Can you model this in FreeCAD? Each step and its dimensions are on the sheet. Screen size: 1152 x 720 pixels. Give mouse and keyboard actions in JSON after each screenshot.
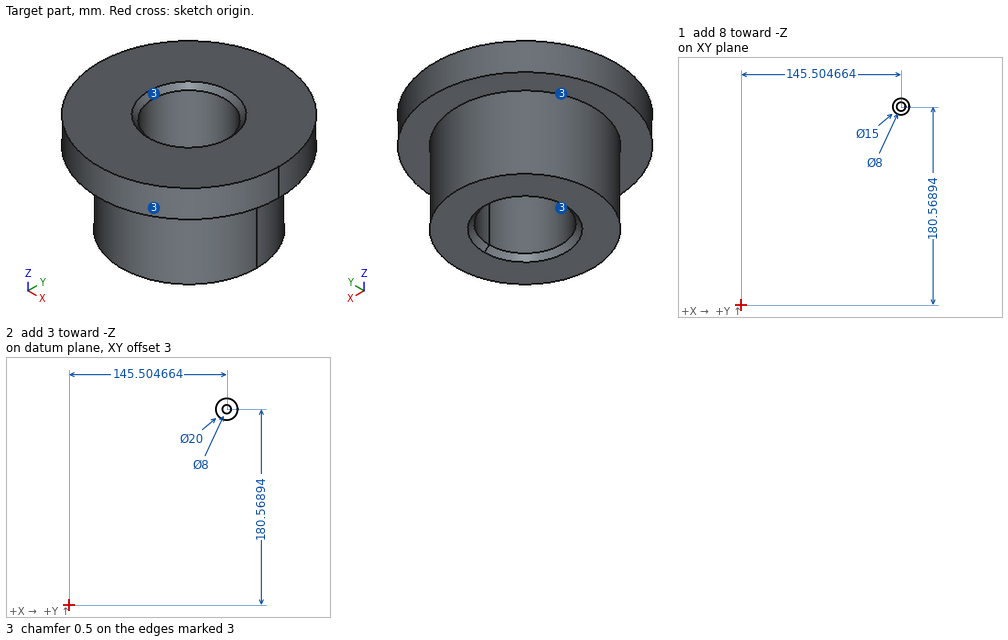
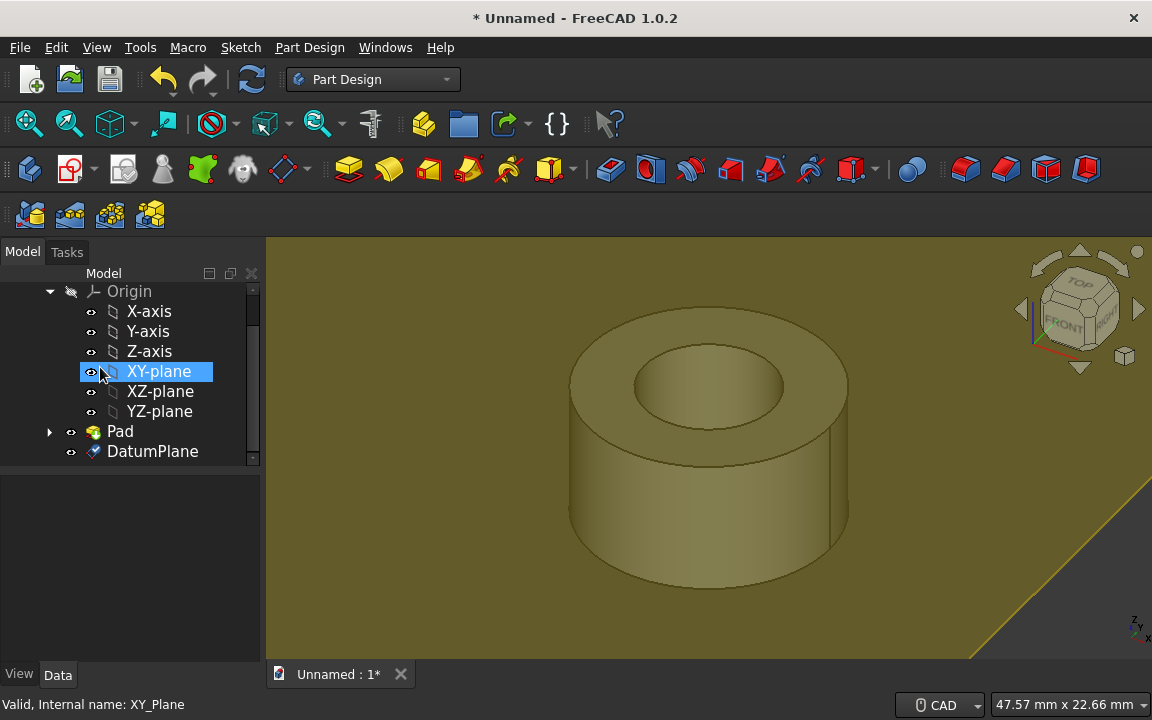
{"action": "left_click", "coordinate": [116, 452]}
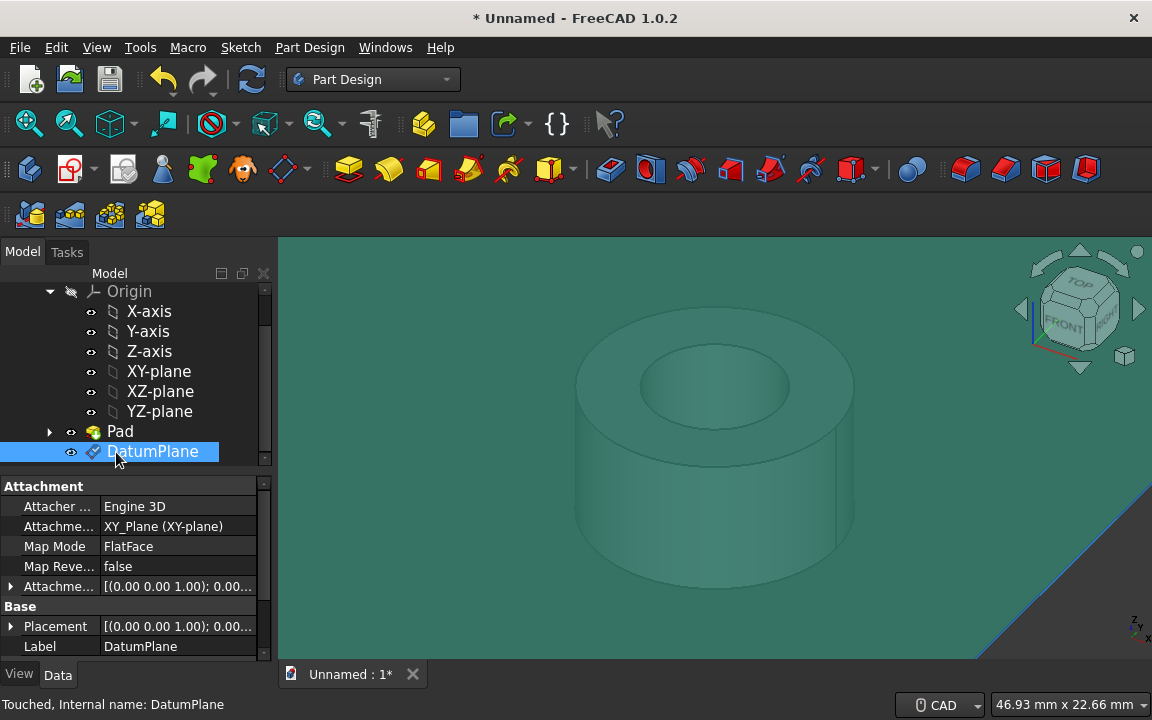
{"action": "left_click", "coordinate": [70, 170]}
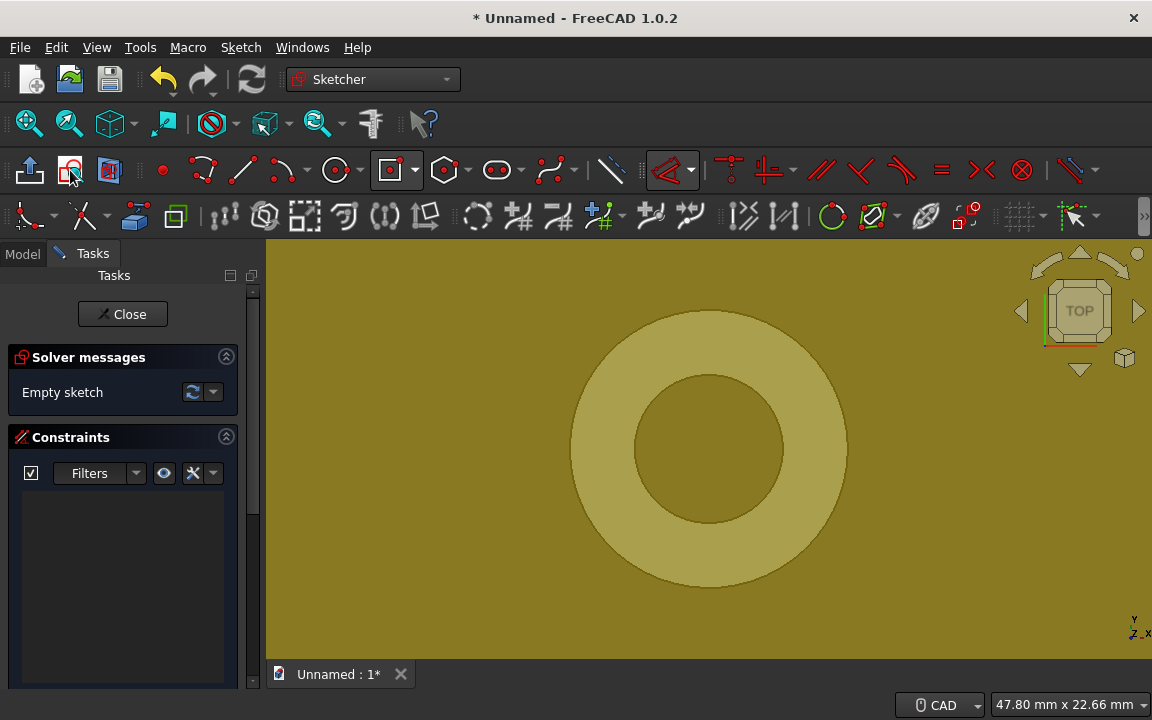
{"action": "scroll", "coordinate": [501, 449], "scroll_direction": "down", "scroll_amount": 2}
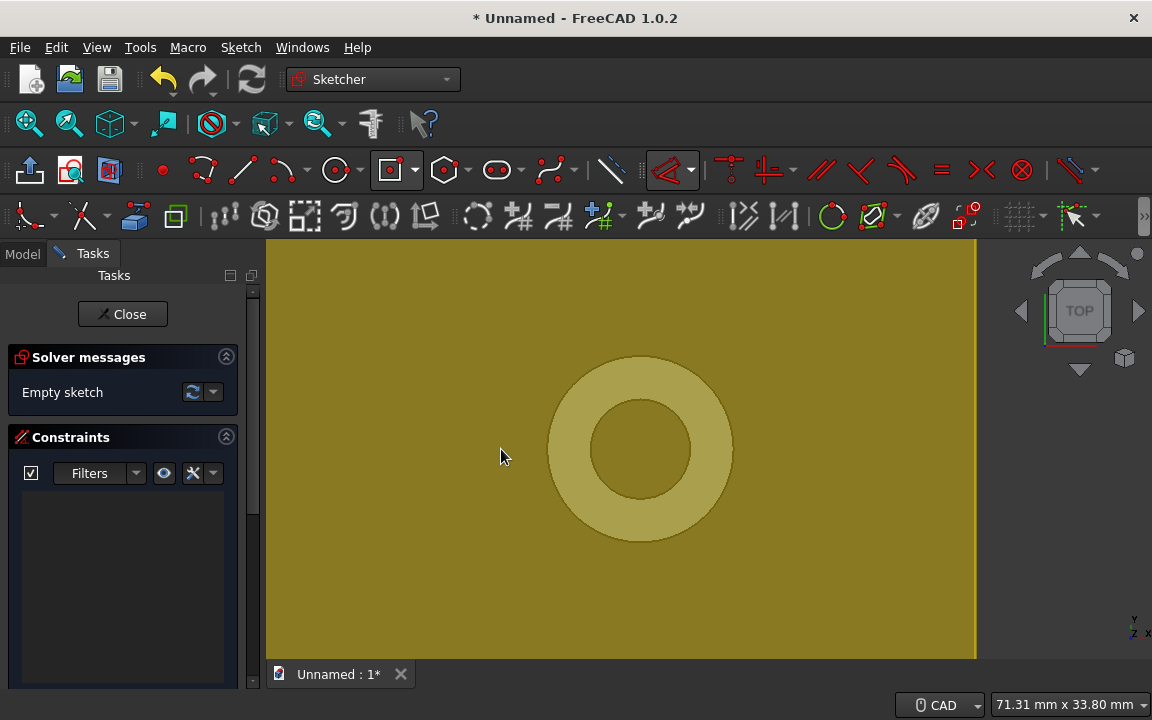
{"action": "key", "text": "g c"}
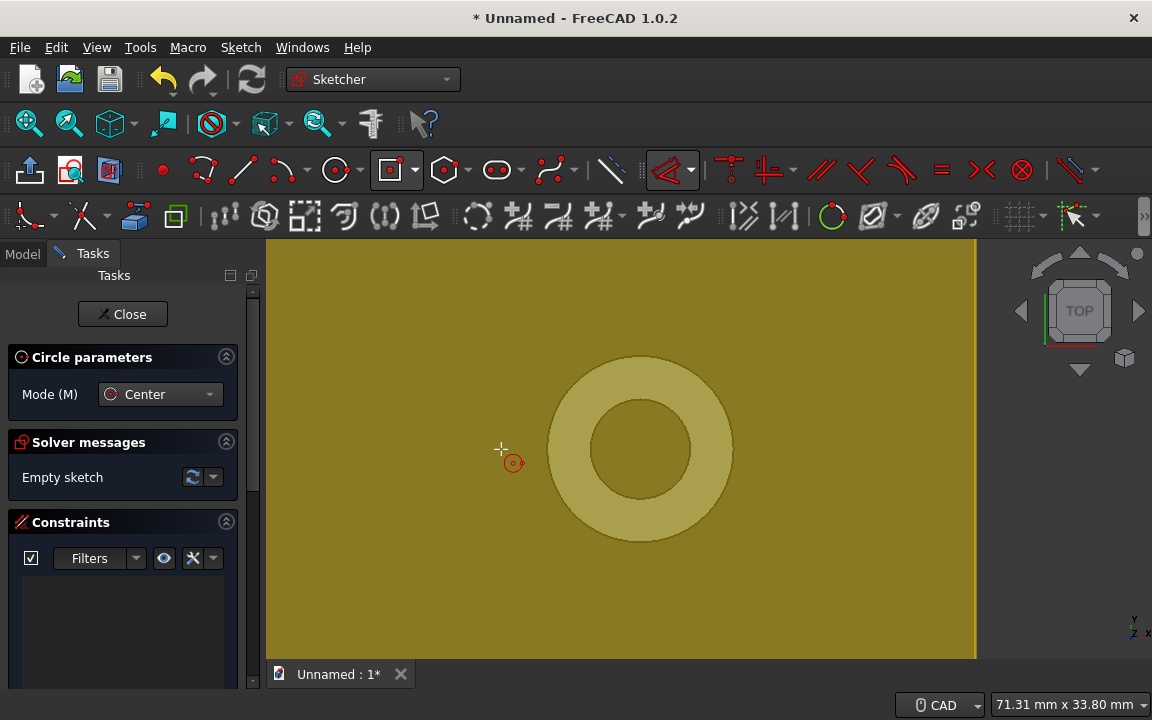
{"action": "left_click", "coordinate": [640, 449]}
{"action": "left_click", "coordinate": [728, 361]}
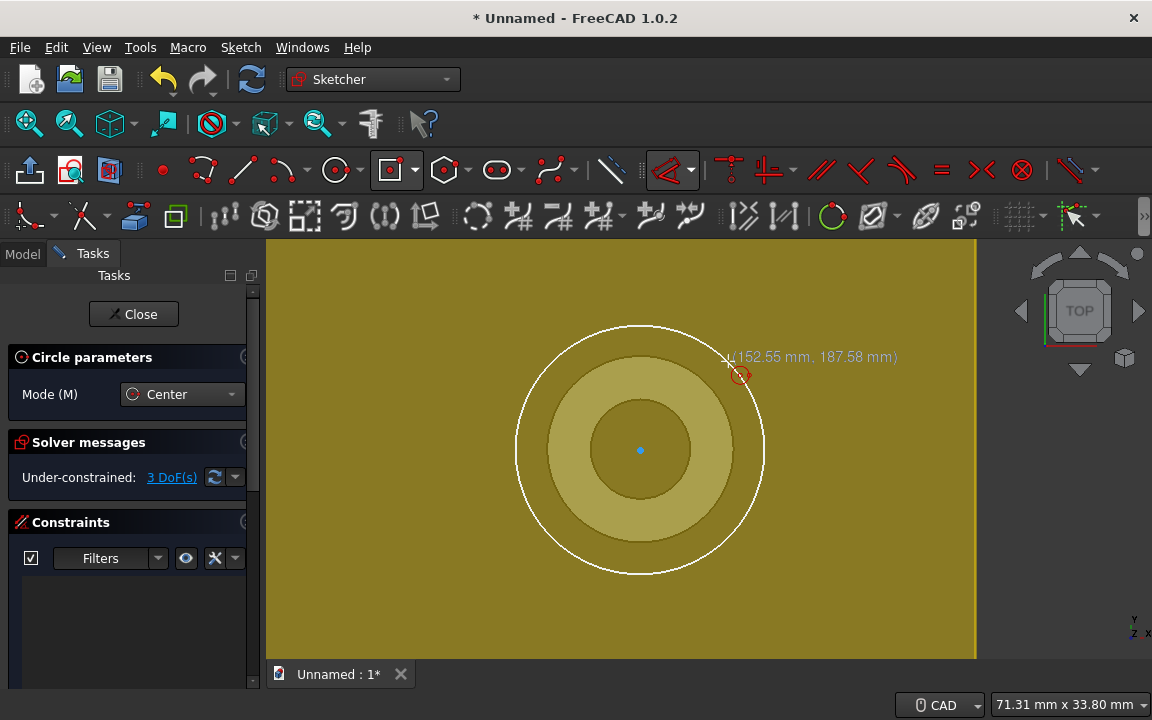
{"action": "left_click", "coordinate": [640, 450]}
{"action": "left_click", "coordinate": [676, 414]}
{"action": "key", "text": "Escape"}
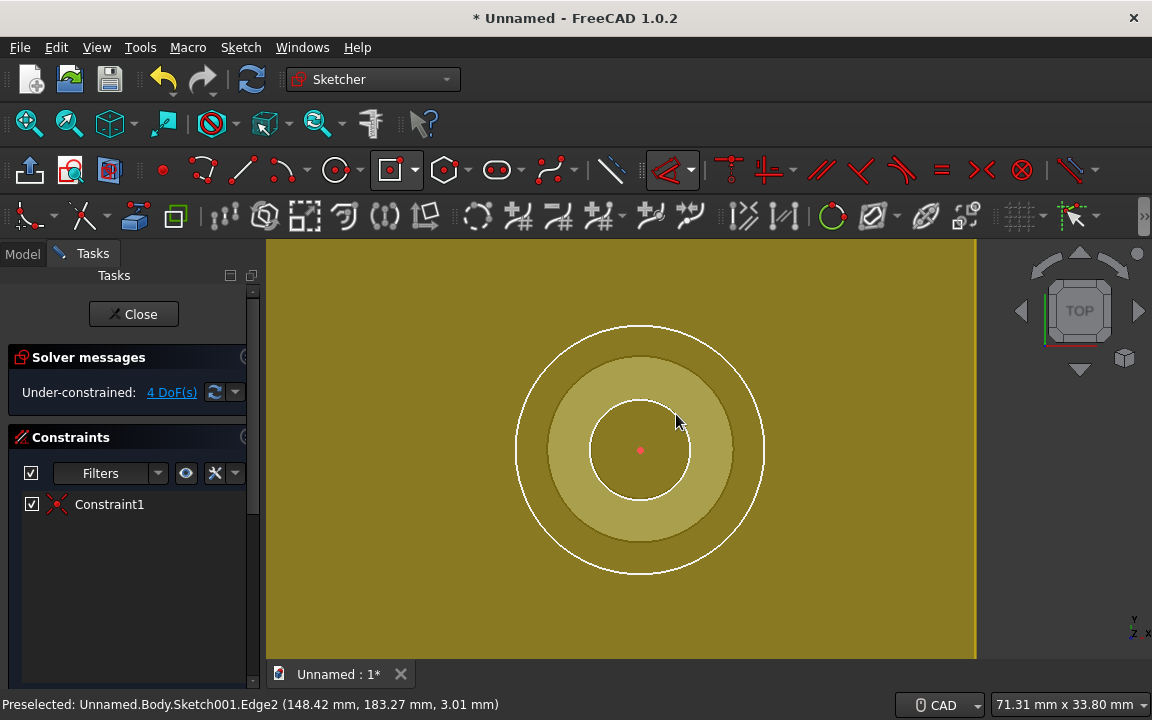
{"action": "key", "text": "d"}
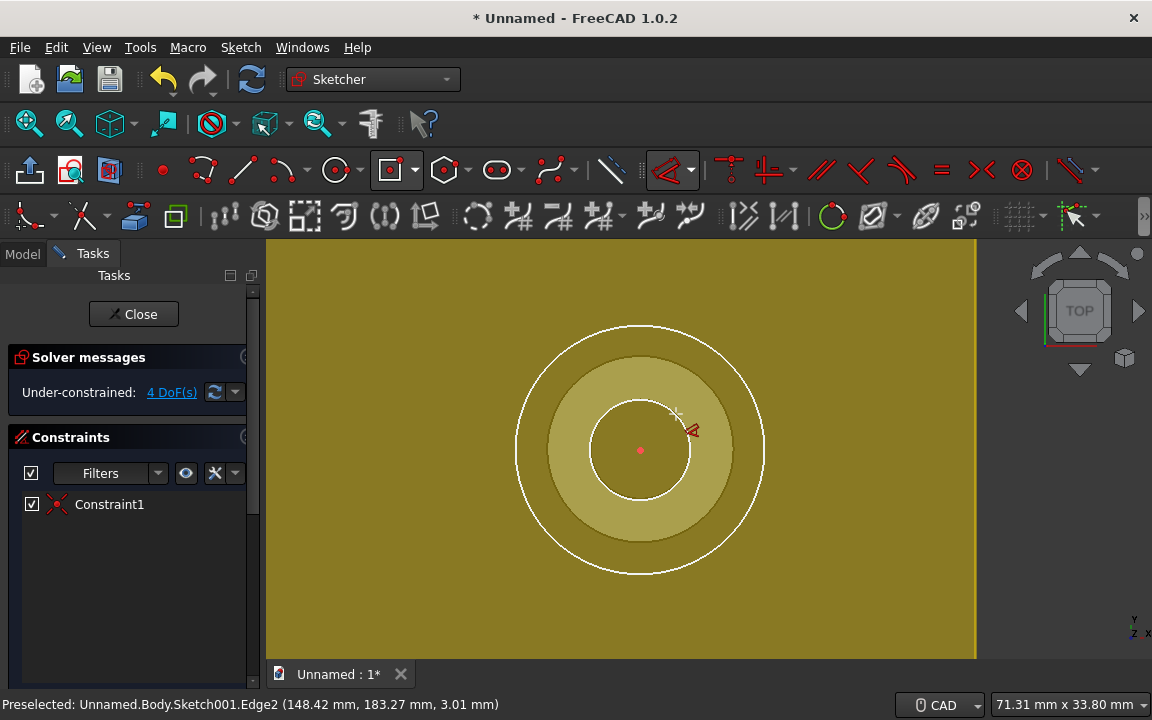
{"action": "left_click", "coordinate": [728, 362]}
{"action": "left_click", "coordinate": [751, 339]}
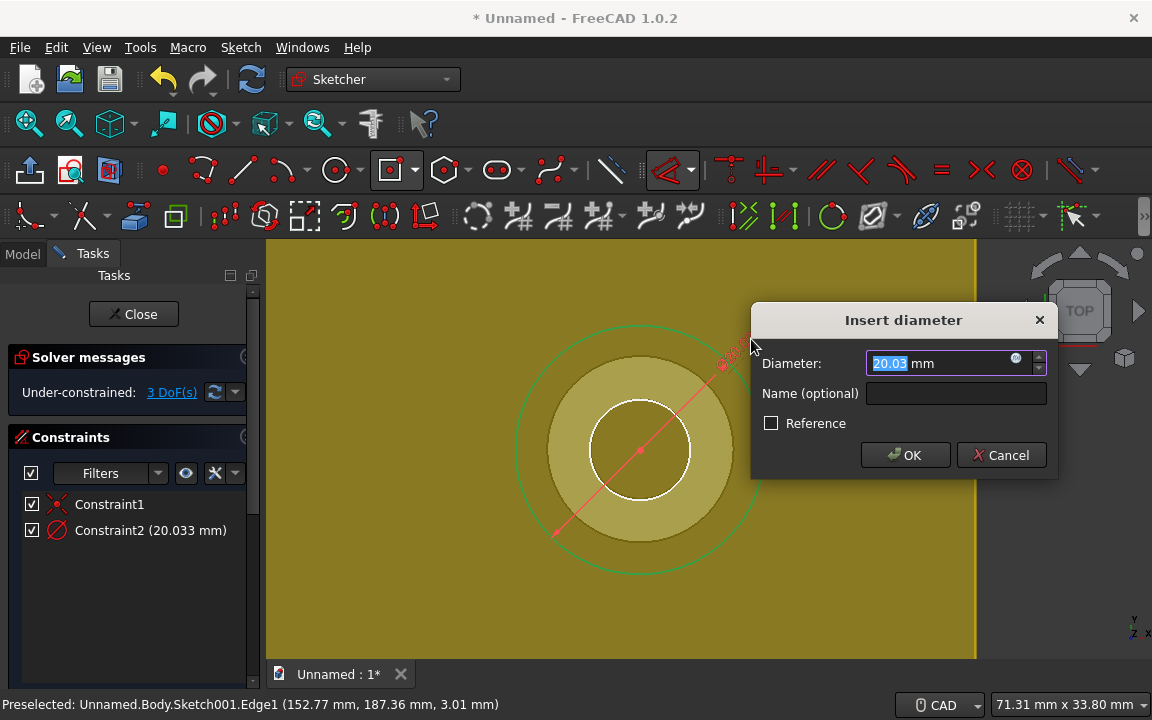
{"action": "type", "text": "20"}
{"action": "key", "text": "Return"}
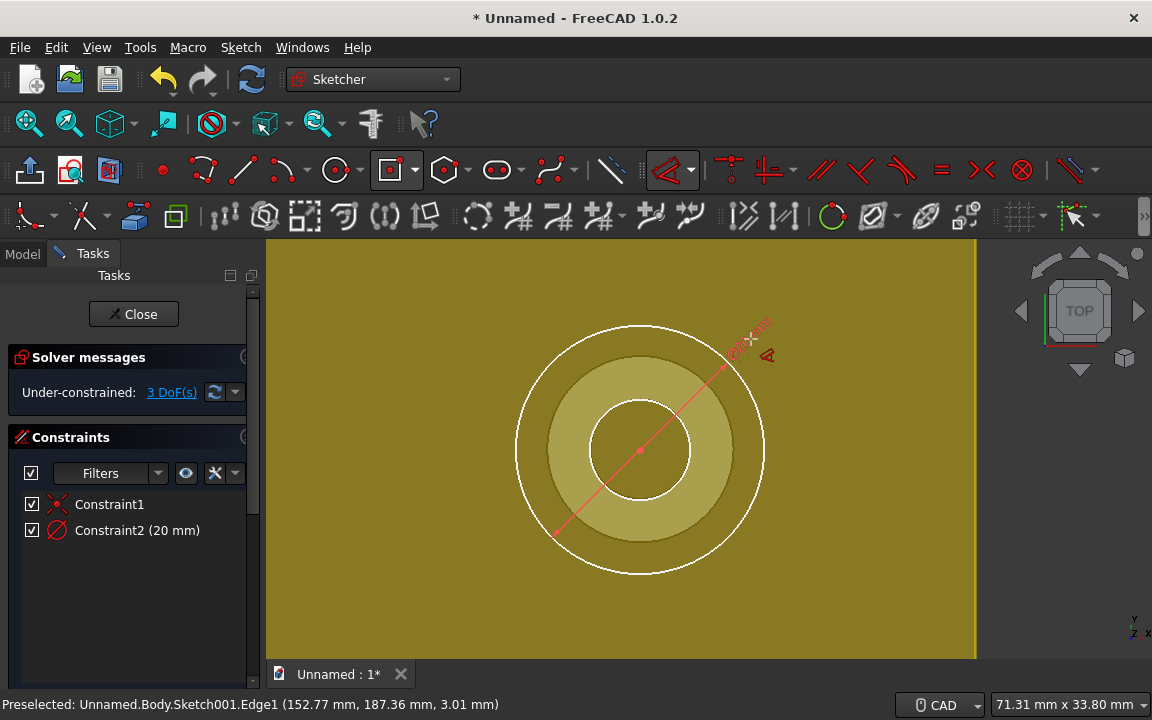
{"action": "left_click", "coordinate": [675, 414]}
{"action": "left_click", "coordinate": [697, 391]}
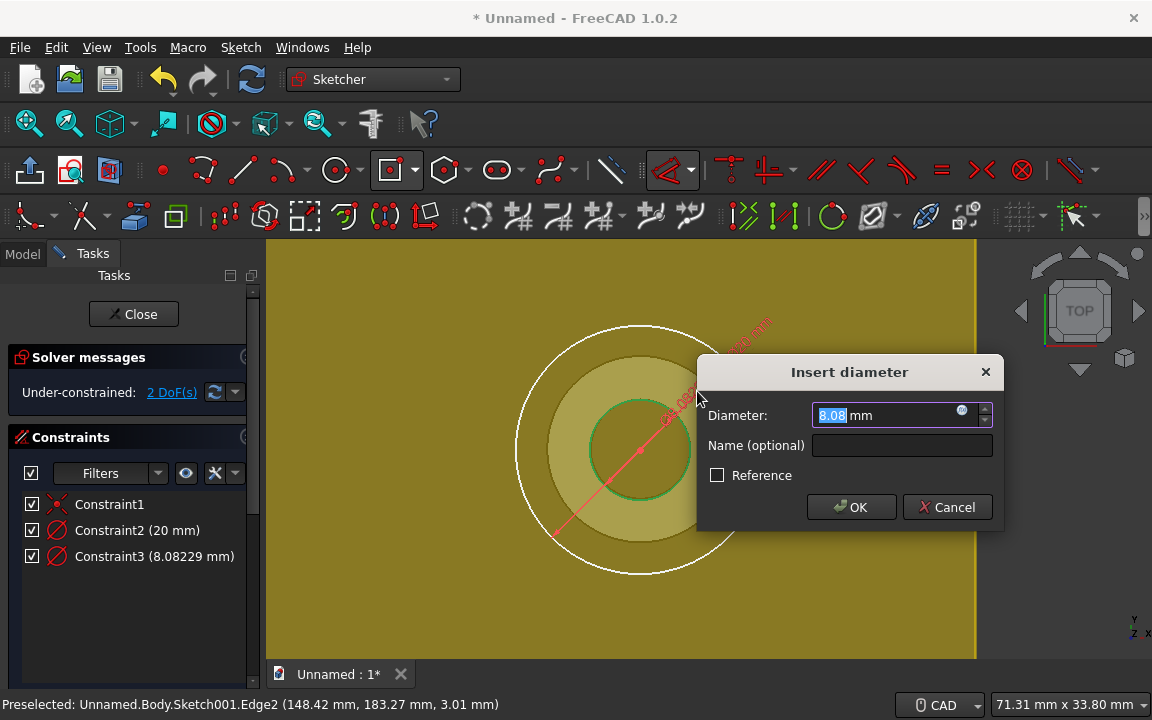
{"action": "type", "text": "8"}
{"action": "key", "text": "Return"}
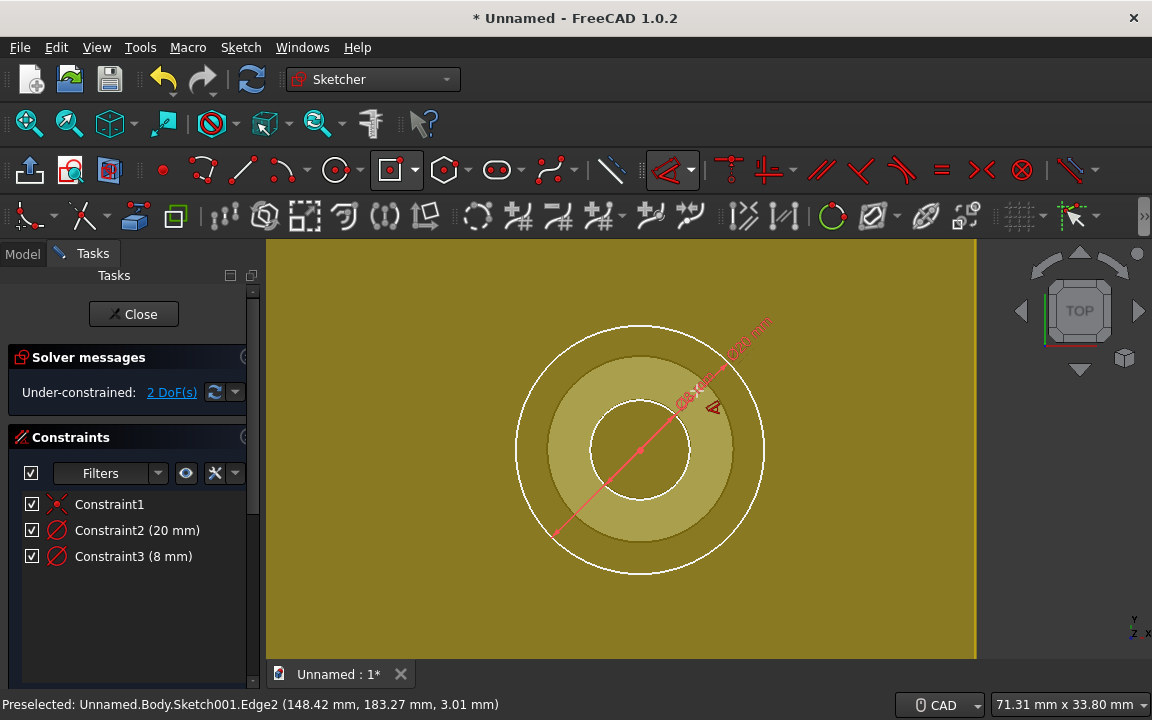
{"action": "left_click", "coordinate": [640, 450]}
{"action": "left_click", "coordinate": [674, 541]}